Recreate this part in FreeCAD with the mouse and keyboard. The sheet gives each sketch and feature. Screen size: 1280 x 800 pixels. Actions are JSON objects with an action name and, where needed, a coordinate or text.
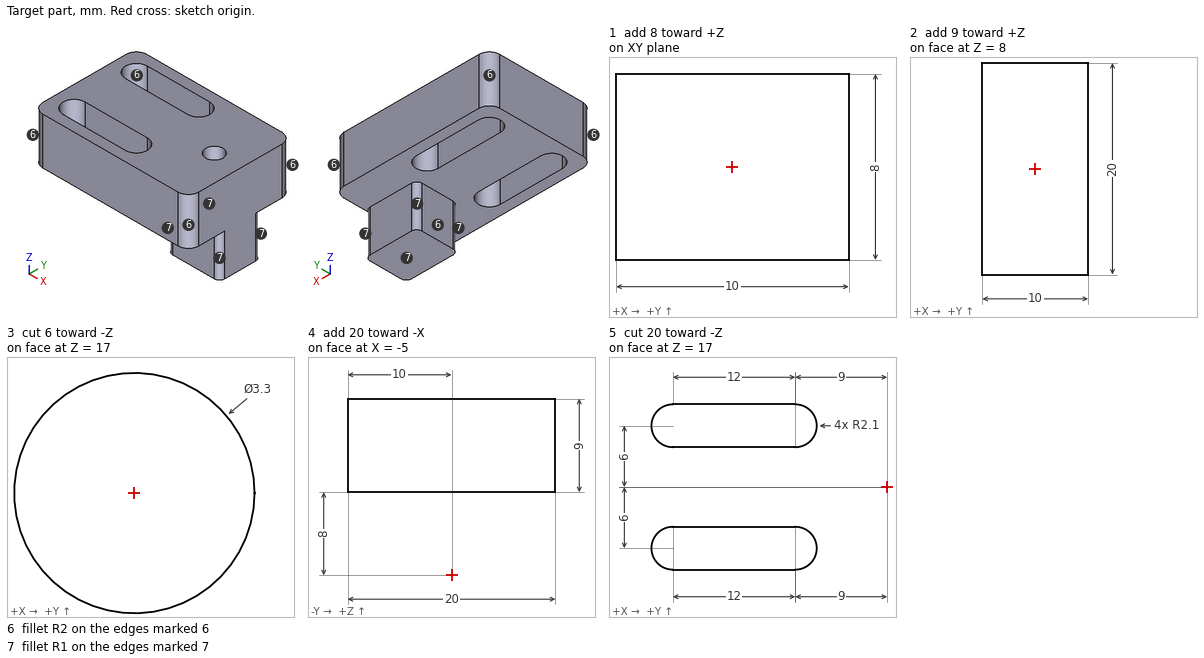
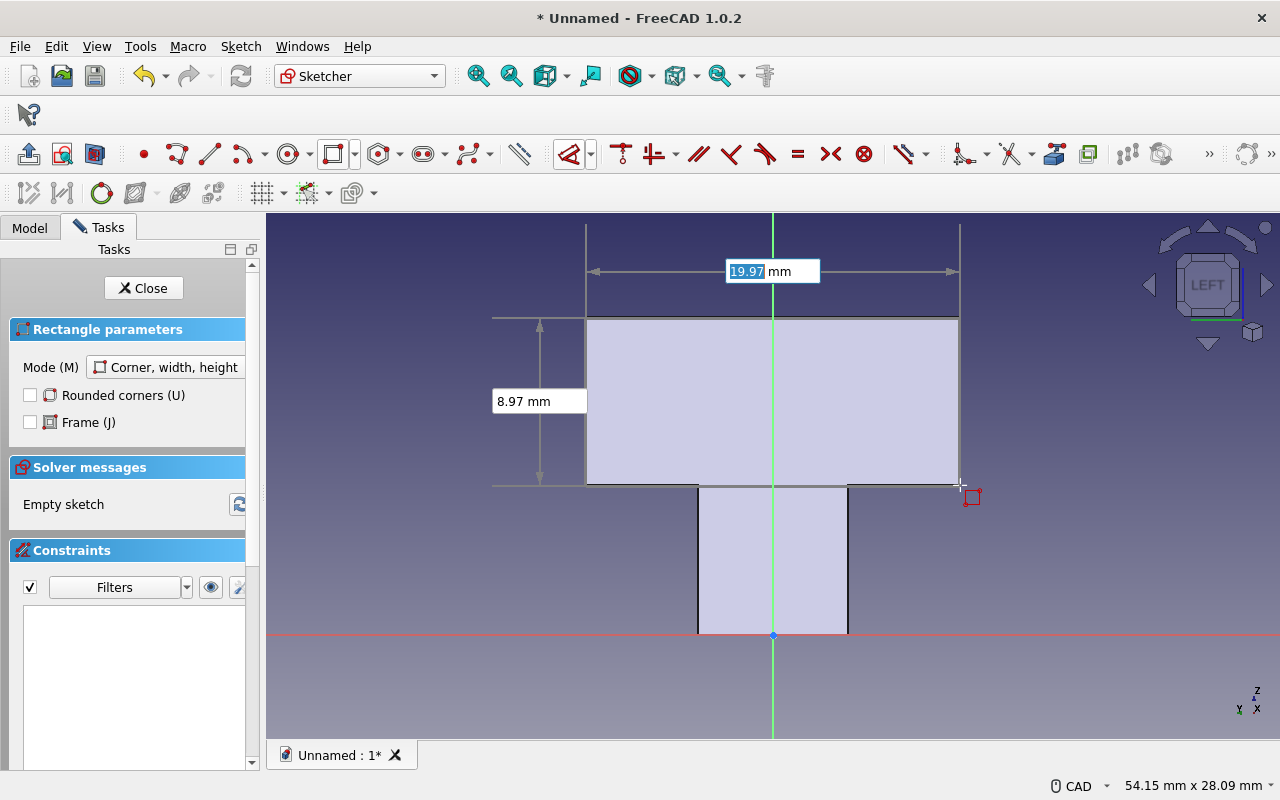
{"action": "type", "text": "20"}
{"action": "key", "text": "Tab"}
{"action": "type", "text": "9"}
{"action": "key", "text": "Return"}
{"action": "key", "text": "Escape"}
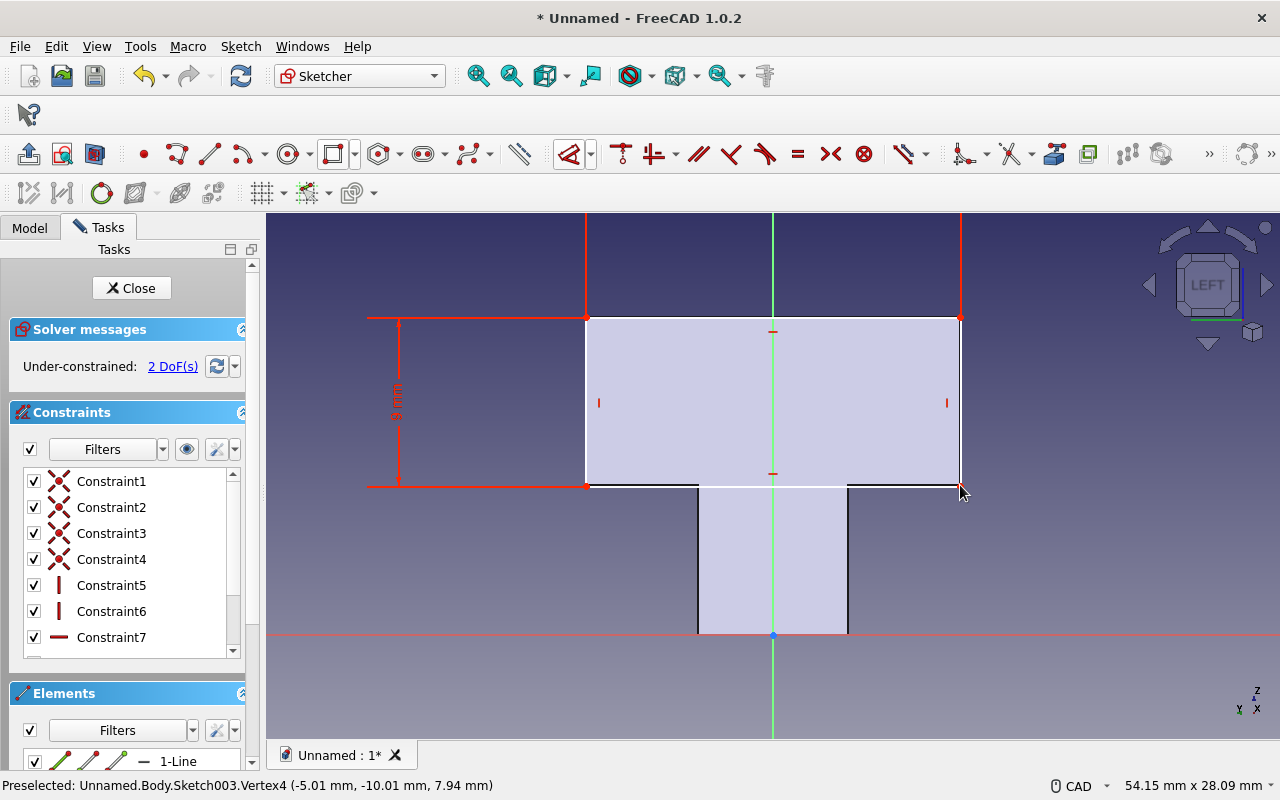
{"action": "left_click", "coordinate": [568, 154]}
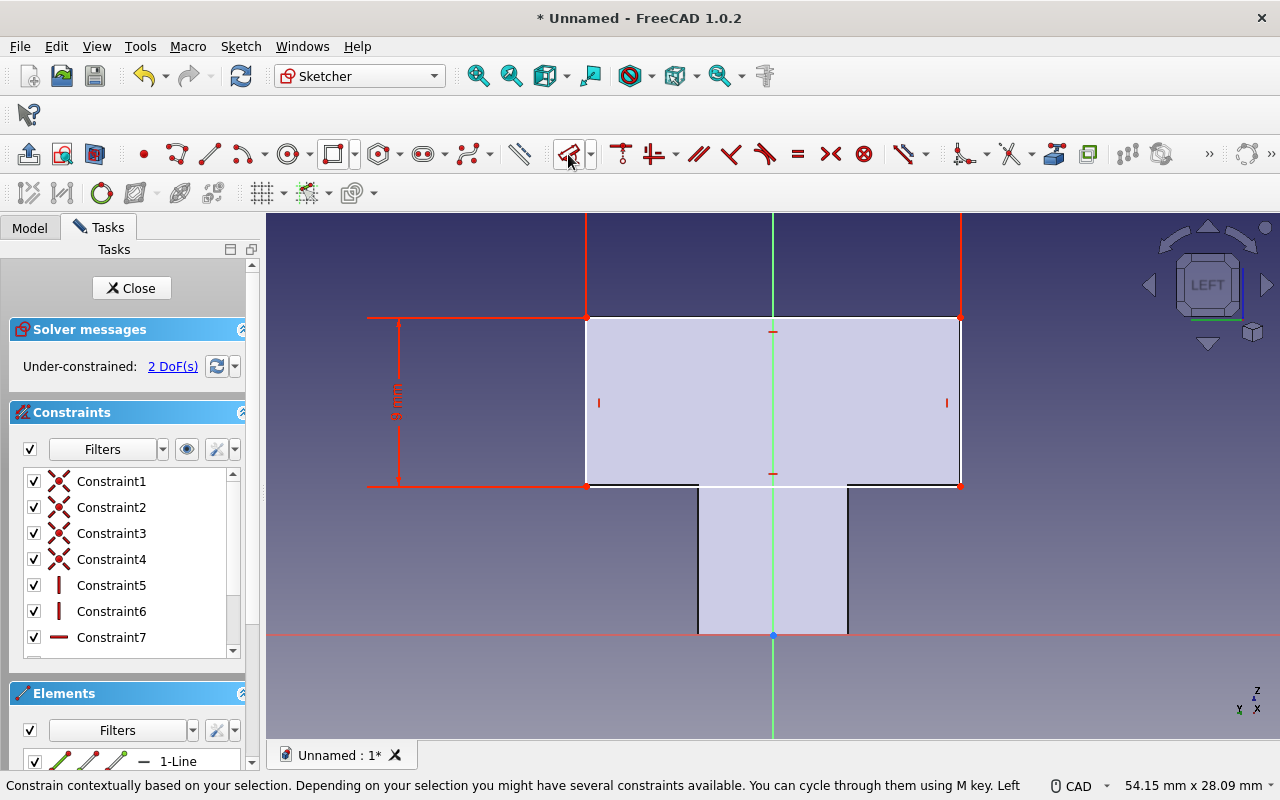
{"action": "left_click", "coordinate": [586, 487]}
{"action": "left_click", "coordinate": [552, 561]}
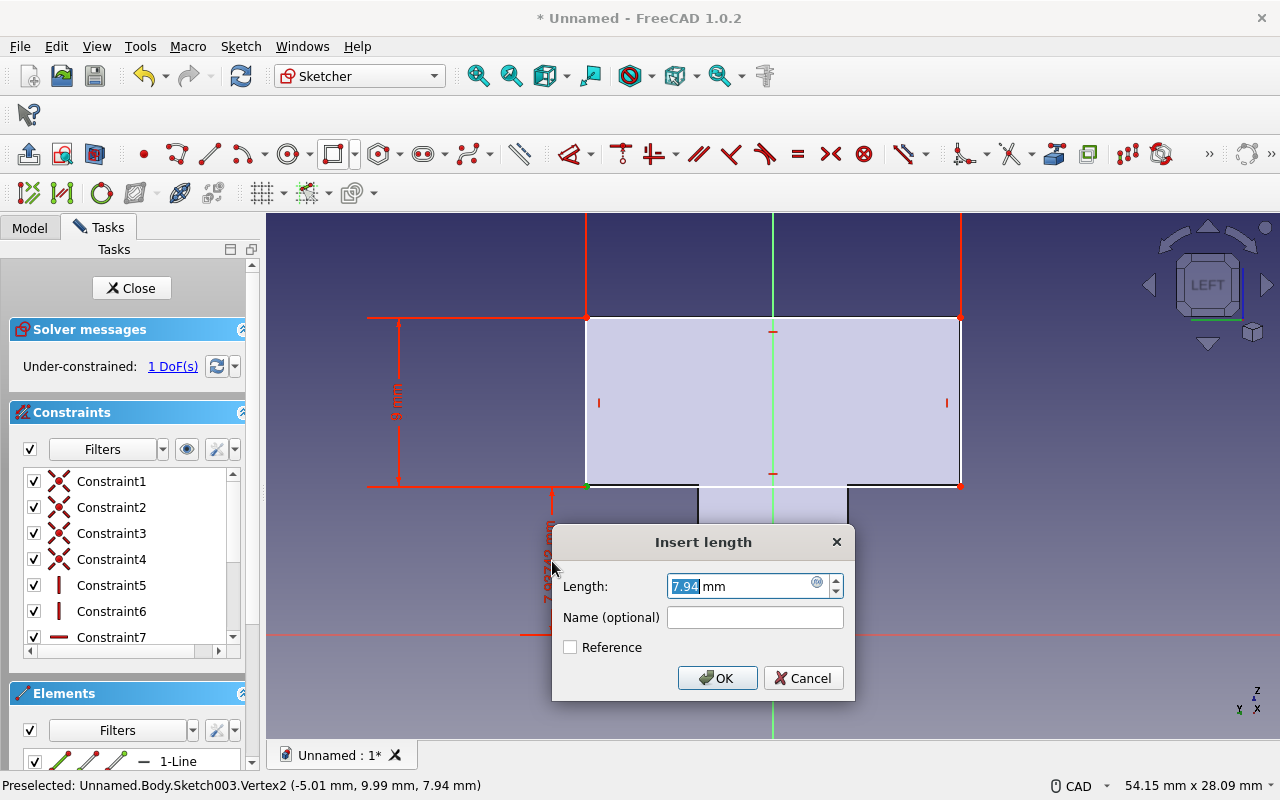
{"action": "type", "text": "8"}
{"action": "key", "text": "Return"}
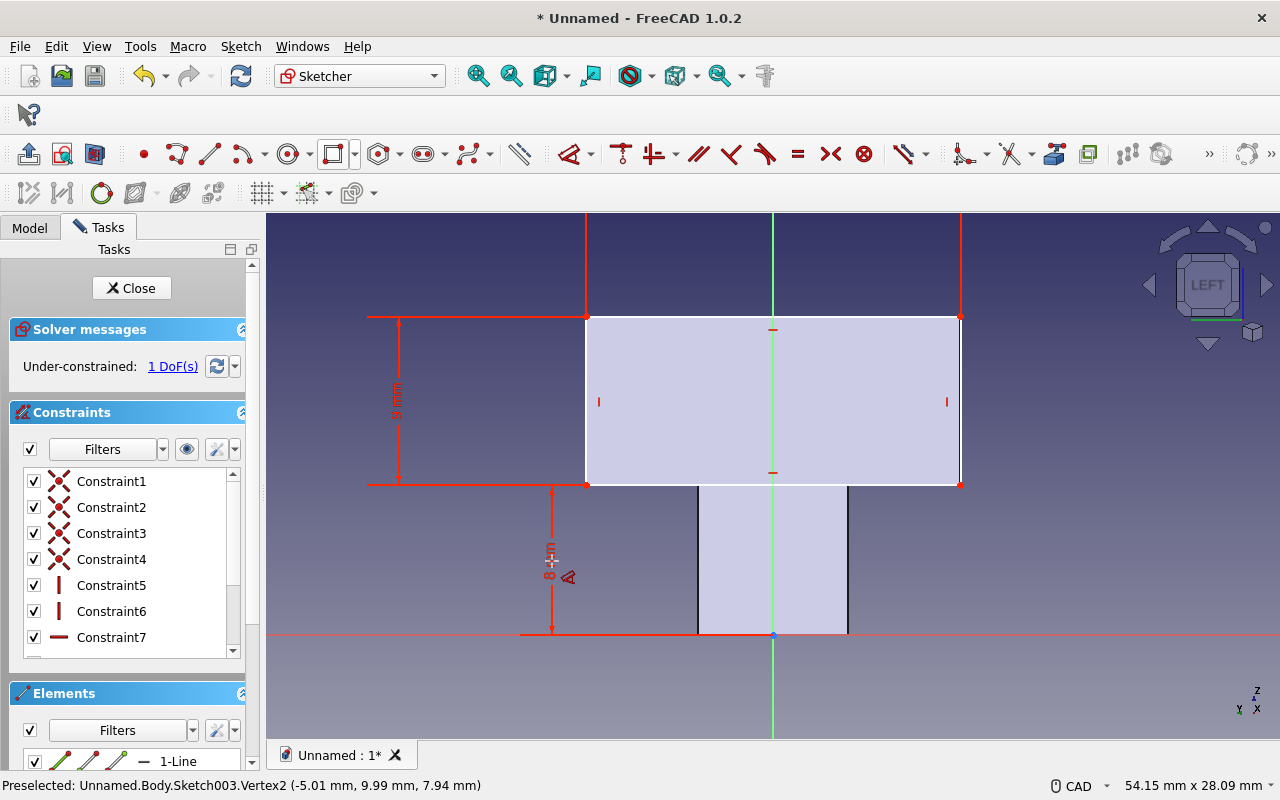
{"action": "left_click", "coordinate": [586, 317]}
{"action": "left_click", "coordinate": [680, 669]}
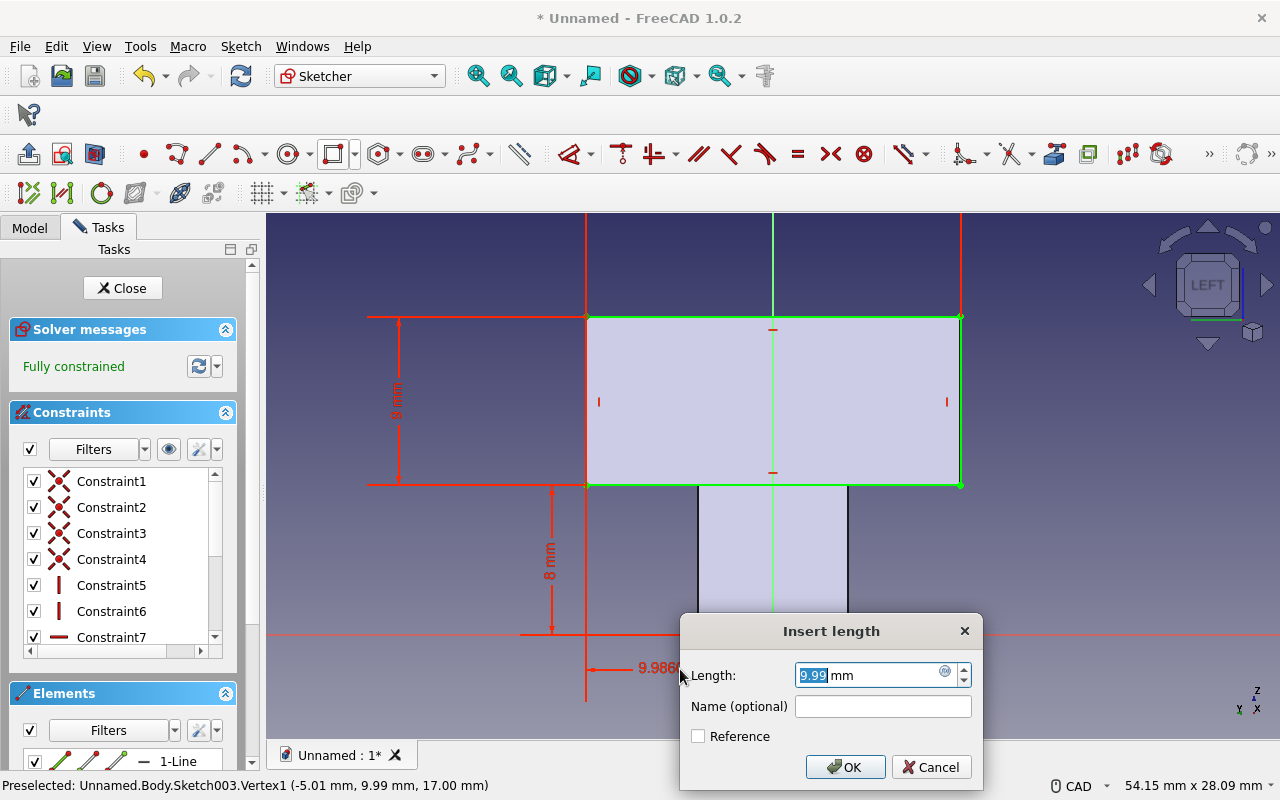
{"action": "type", "text": "10"}
{"action": "key", "text": "Return"}
{"action": "key", "text": "Escape"}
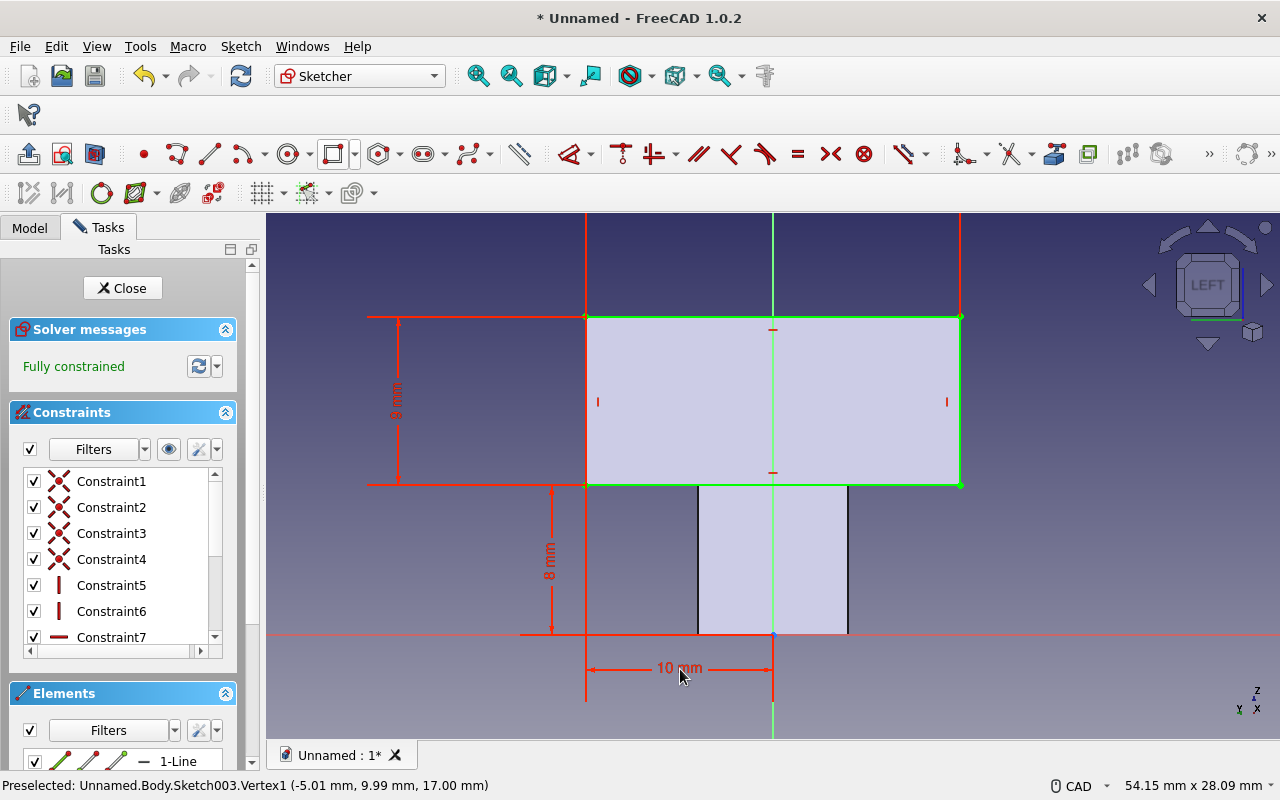
{"action": "left_click", "coordinate": [123, 288]}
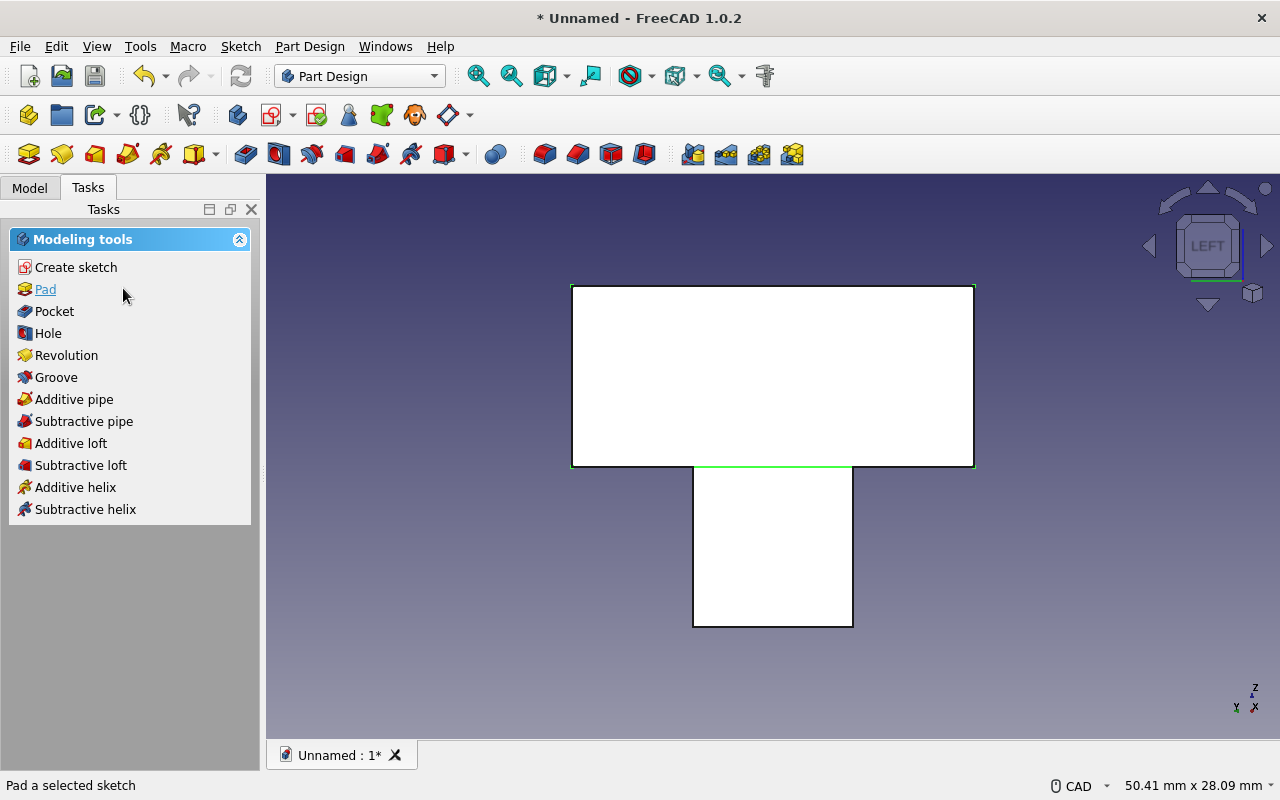
{"action": "left_click", "coordinate": [29, 154]}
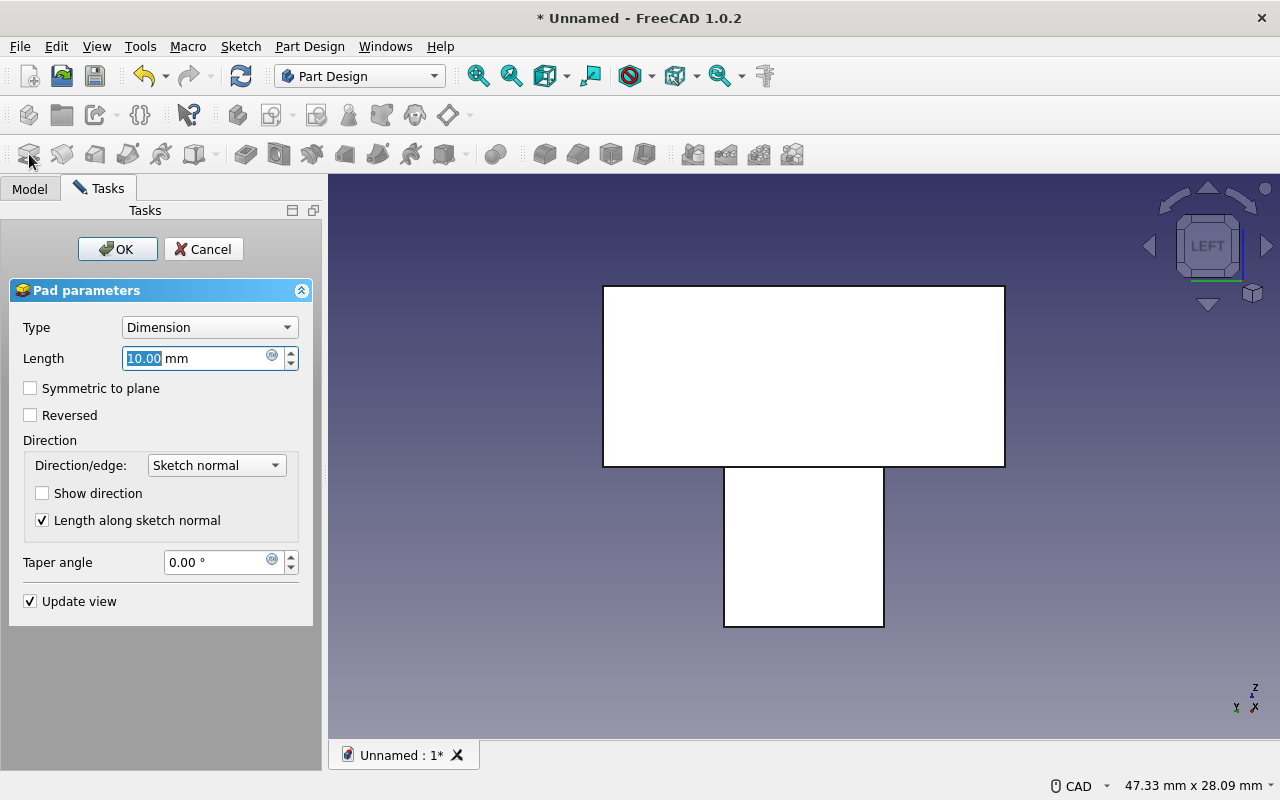
{"action": "type", "text": "20"}
{"action": "key", "text": "Tab"}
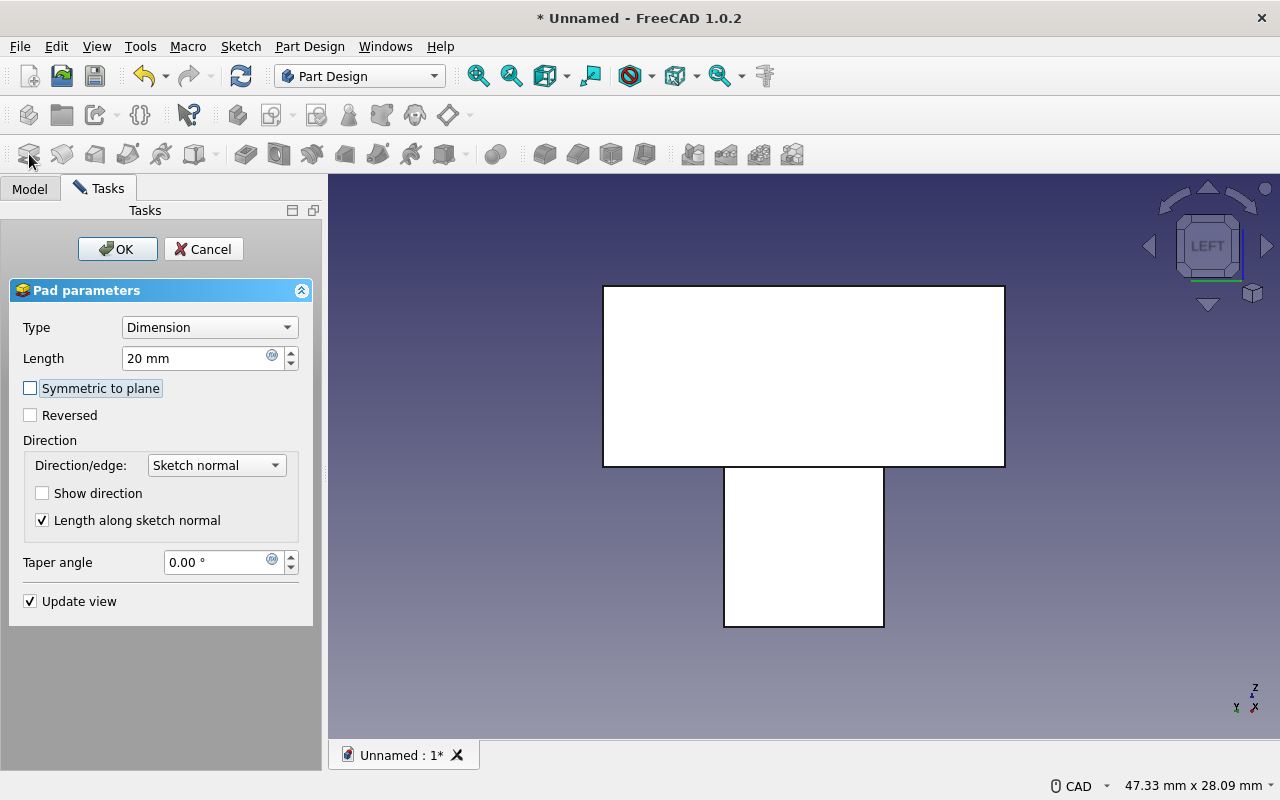
{"action": "left_click", "coordinate": [118, 249]}